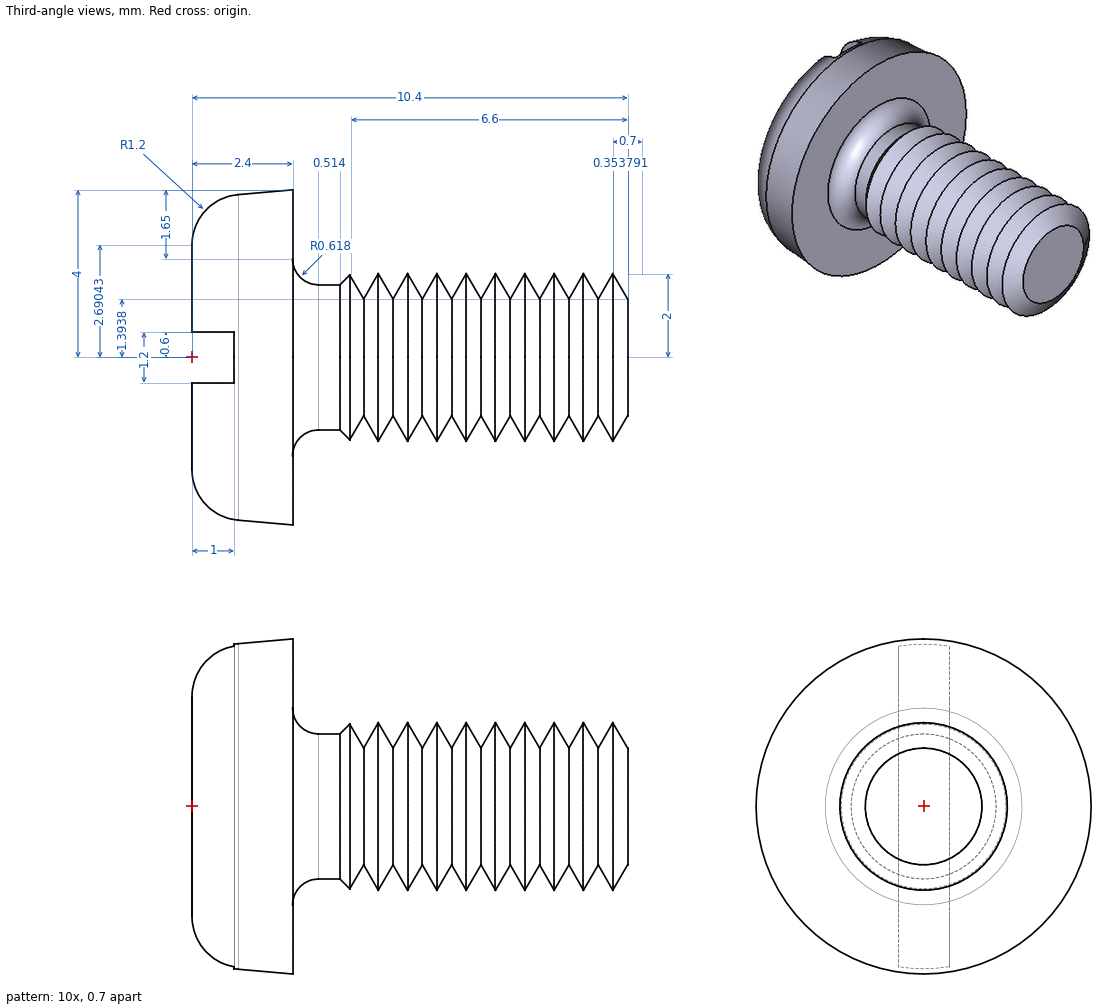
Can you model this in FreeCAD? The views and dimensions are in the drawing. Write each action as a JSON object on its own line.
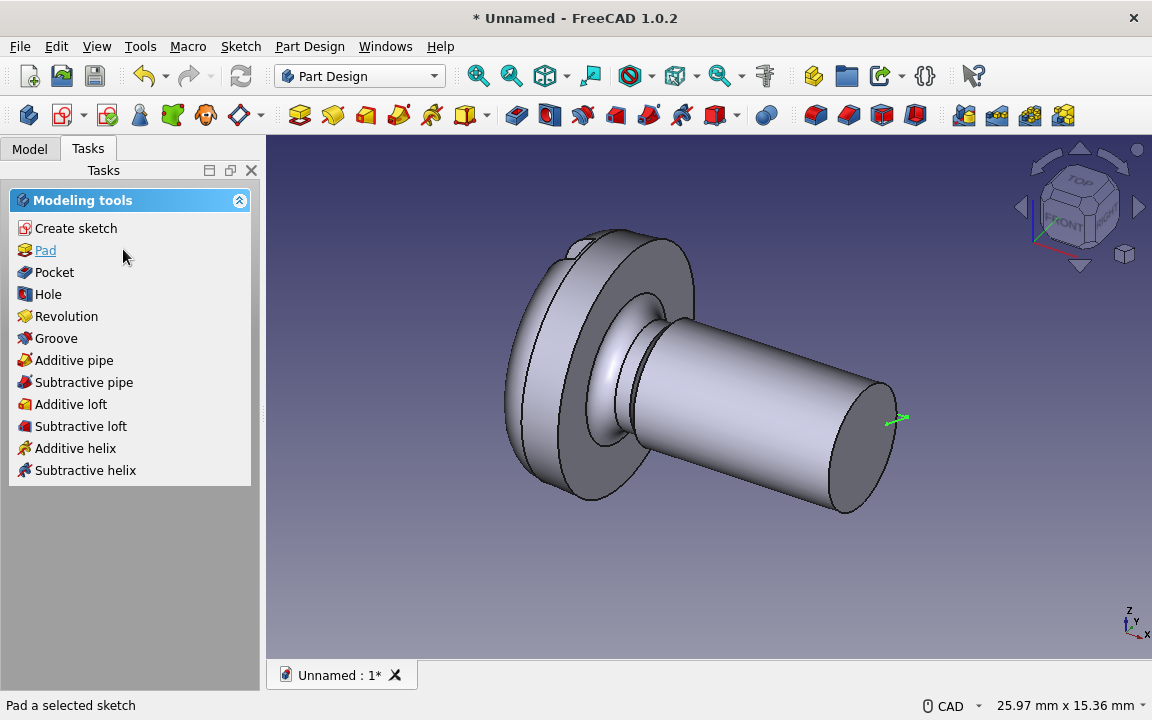
{"action": "left_click", "coordinate": [583, 116]}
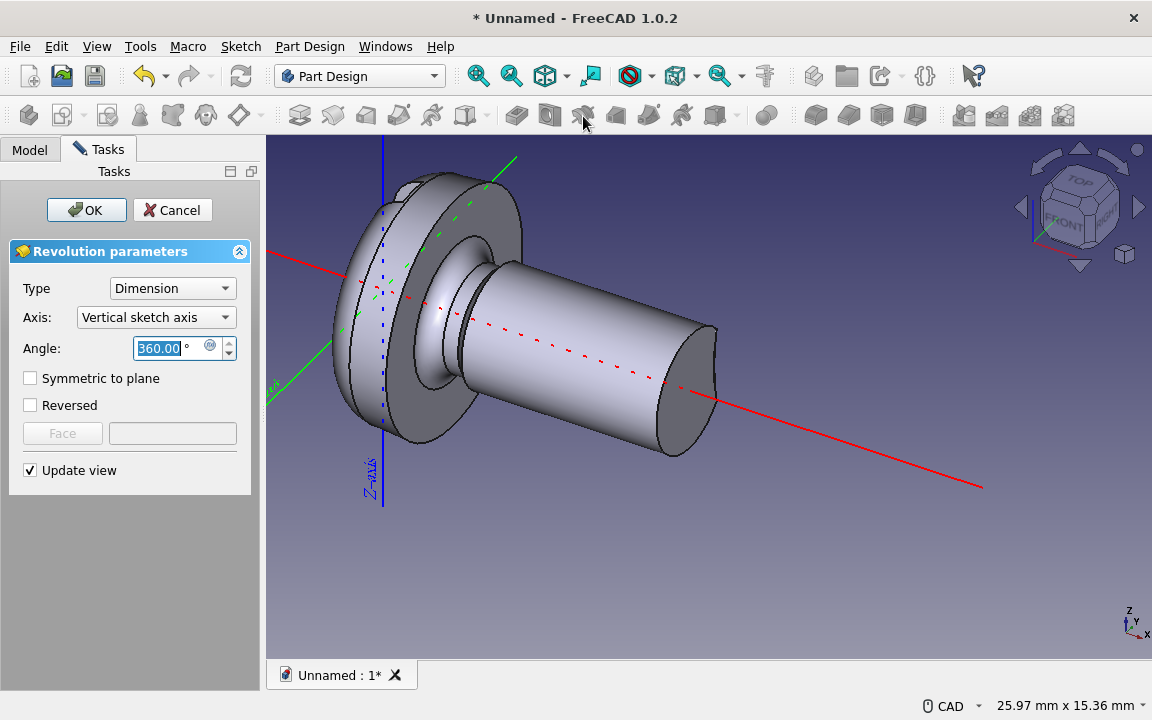
{"action": "left_click", "coordinate": [157, 318]}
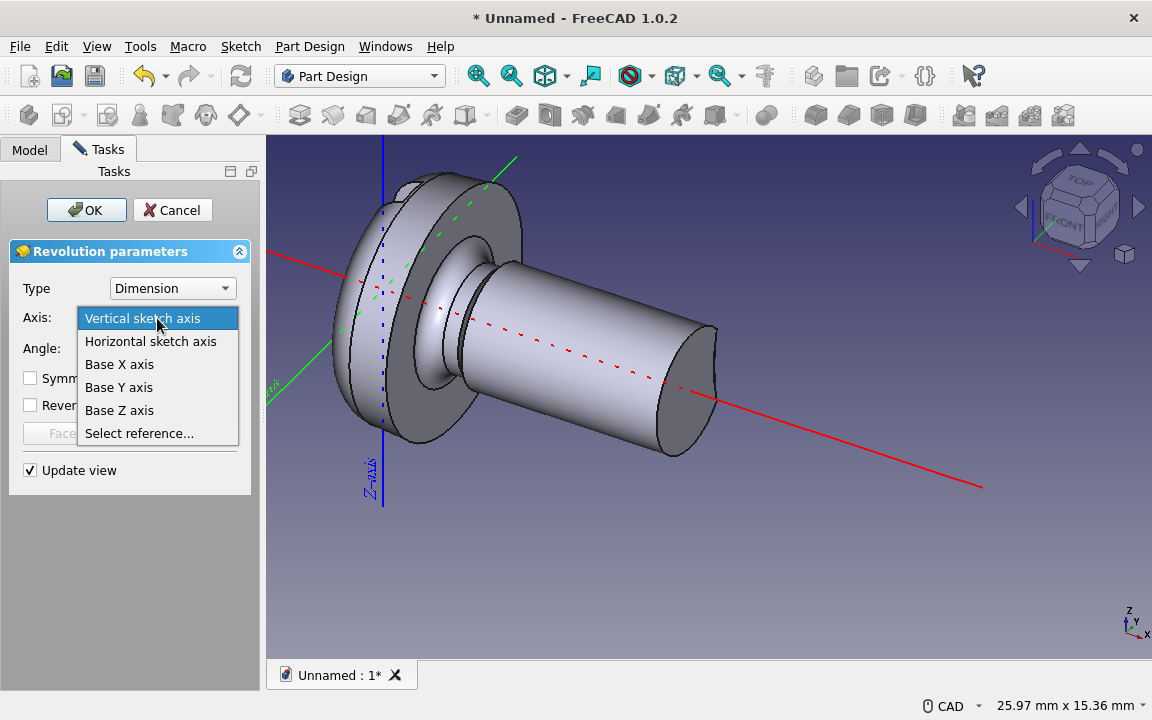
{"action": "left_click", "coordinate": [156, 342]}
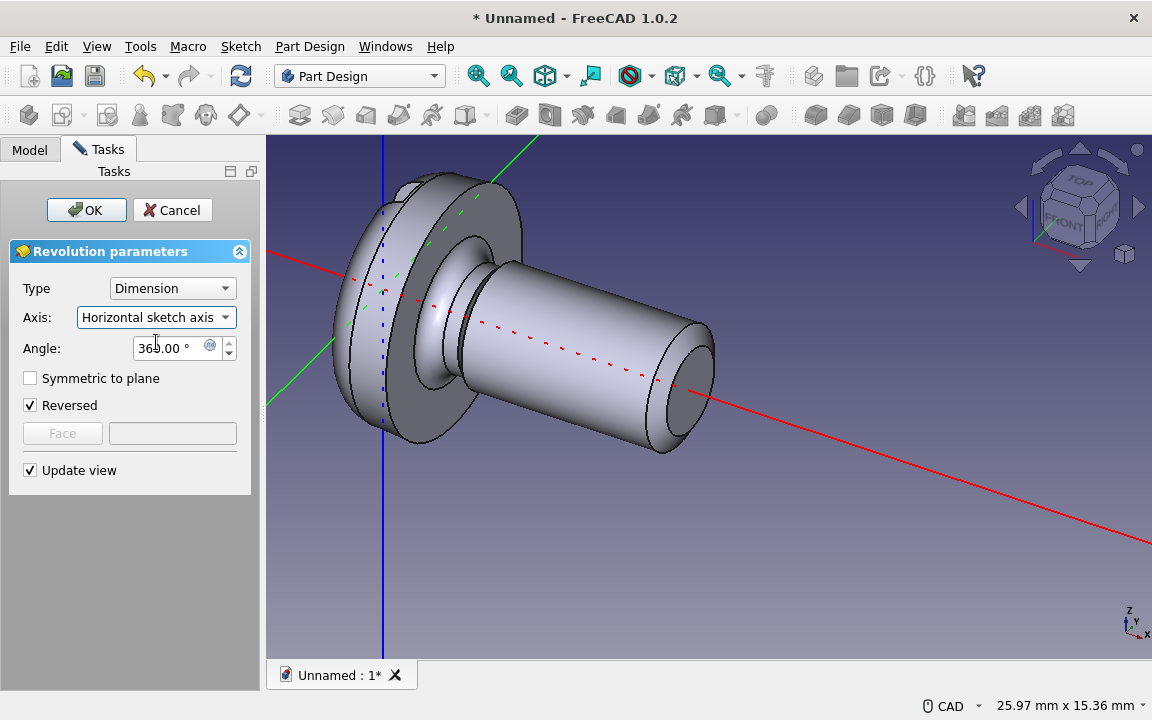
{"action": "left_click", "coordinate": [87, 210]}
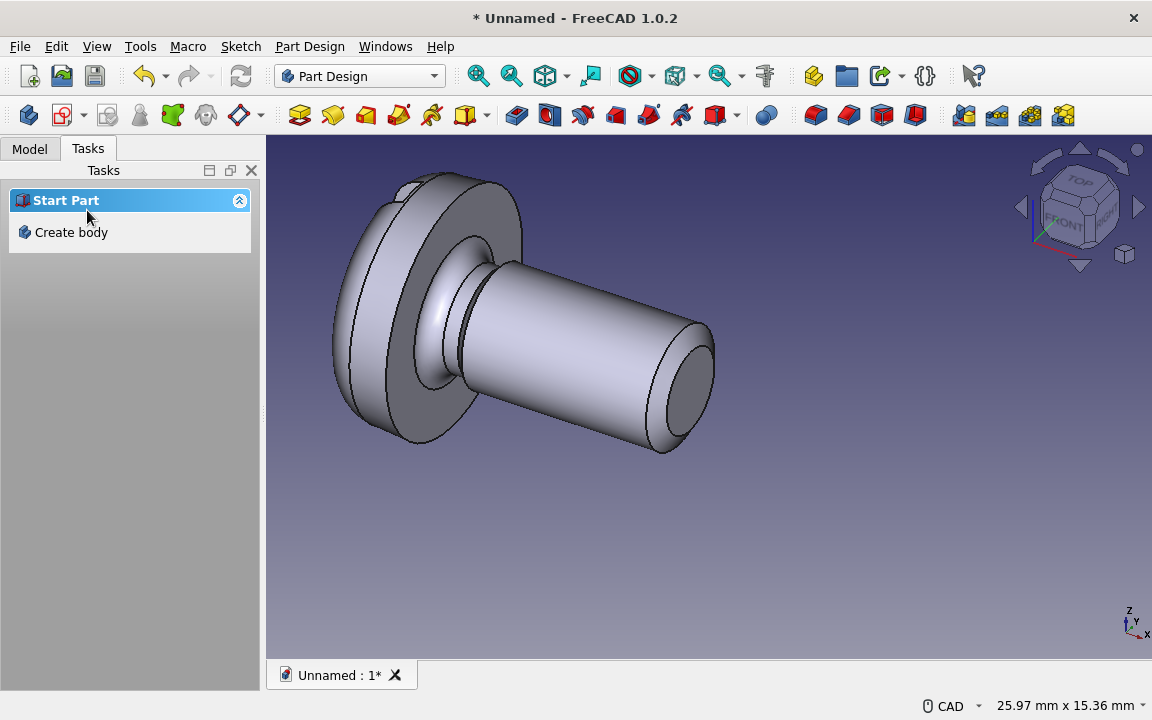
{"action": "left_click", "coordinate": [479, 76]}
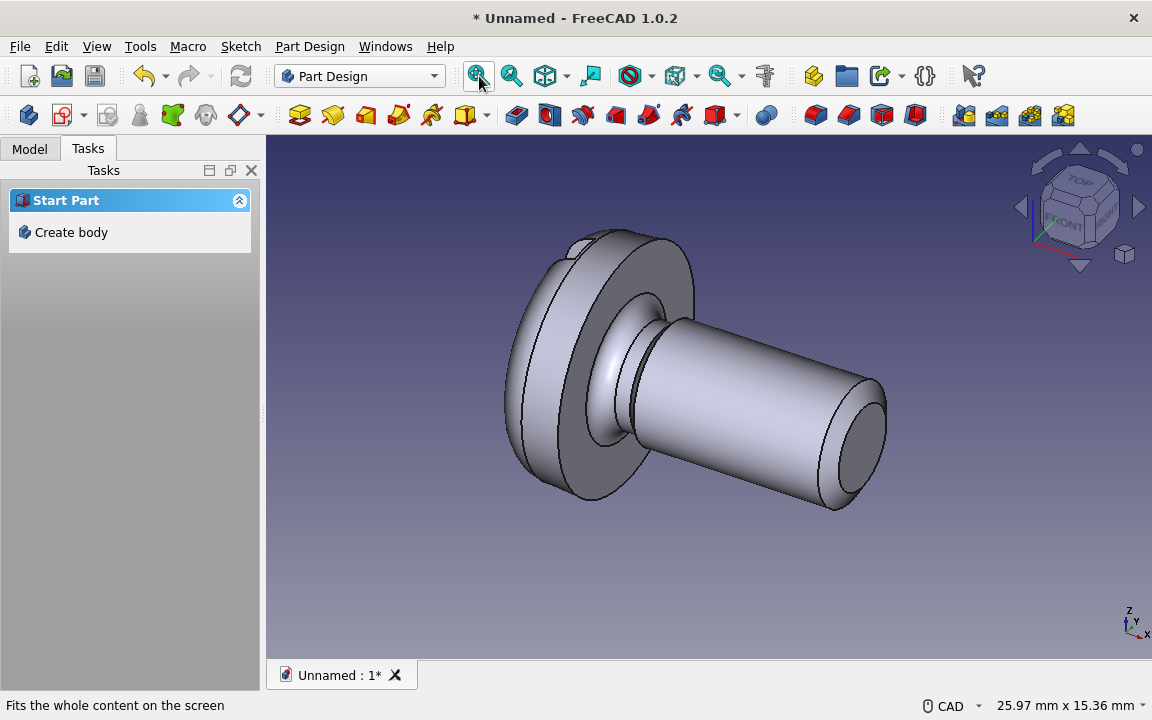
{"action": "left_click", "coordinate": [30, 148]}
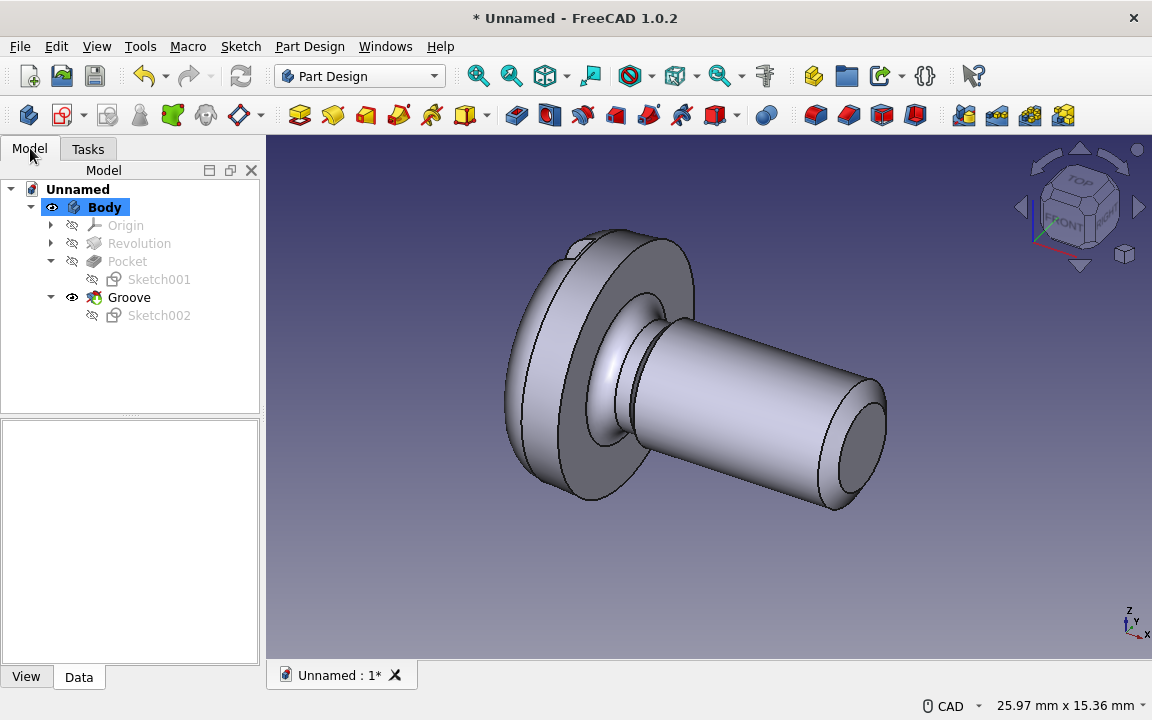
{"action": "left_click", "coordinate": [117, 297]}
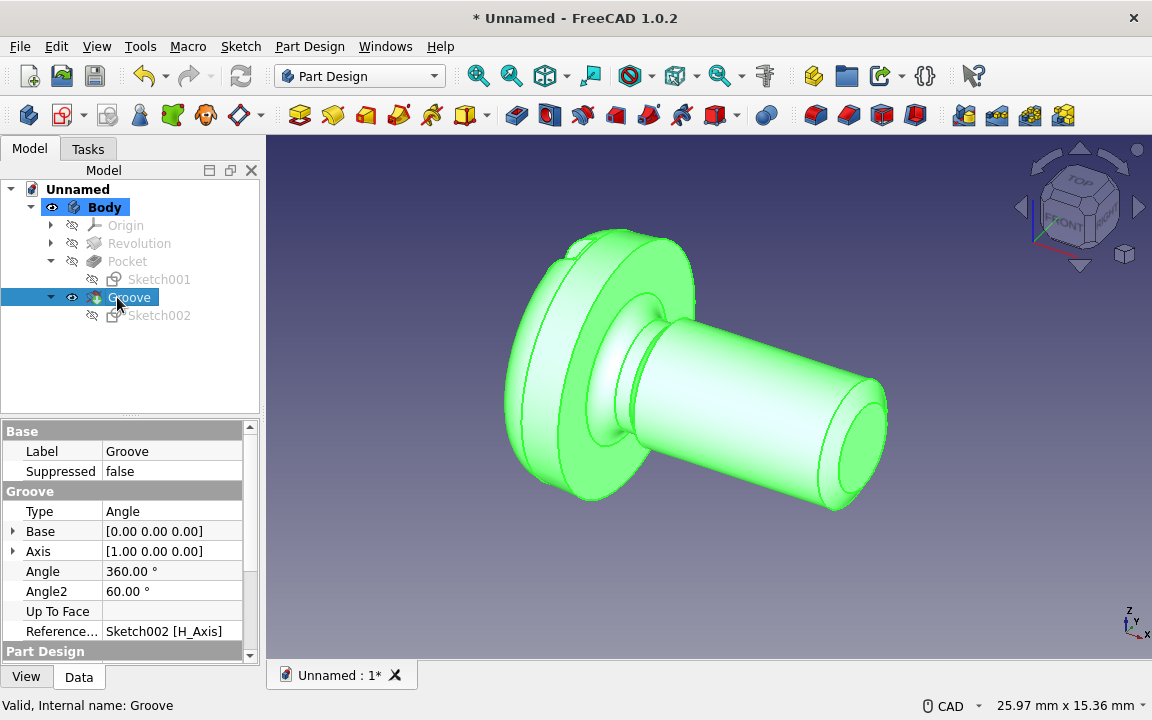
{"action": "left_click", "coordinate": [997, 116]}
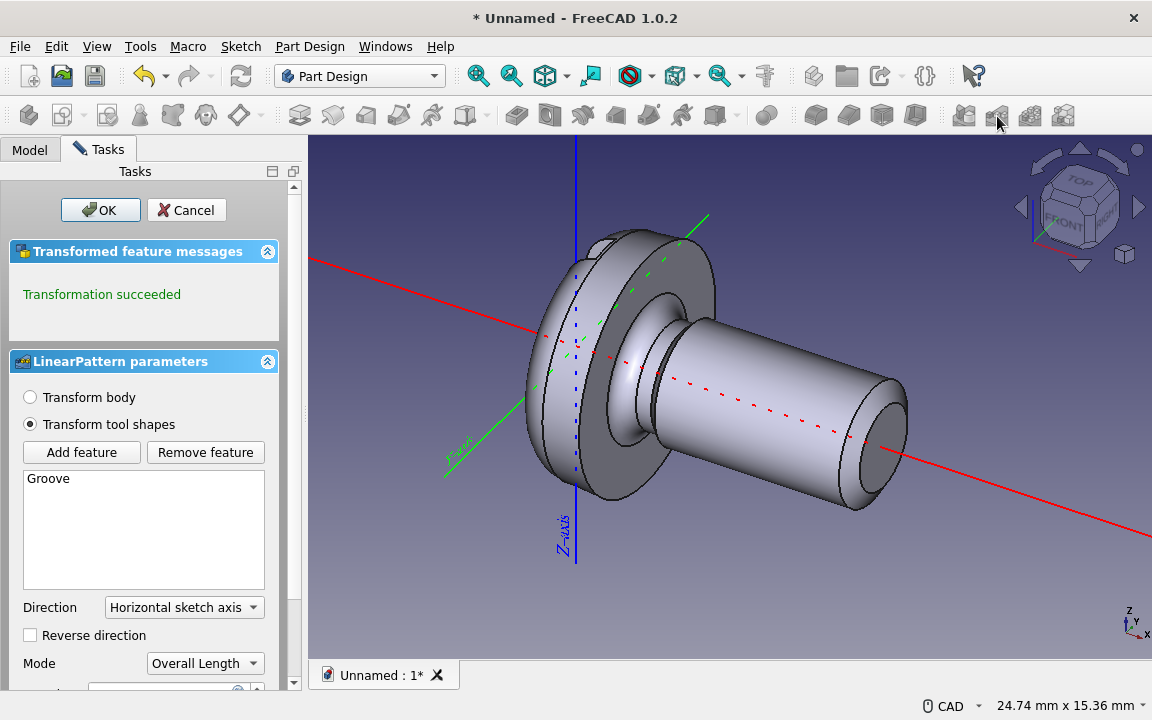
{"action": "left_click", "coordinate": [185, 608]}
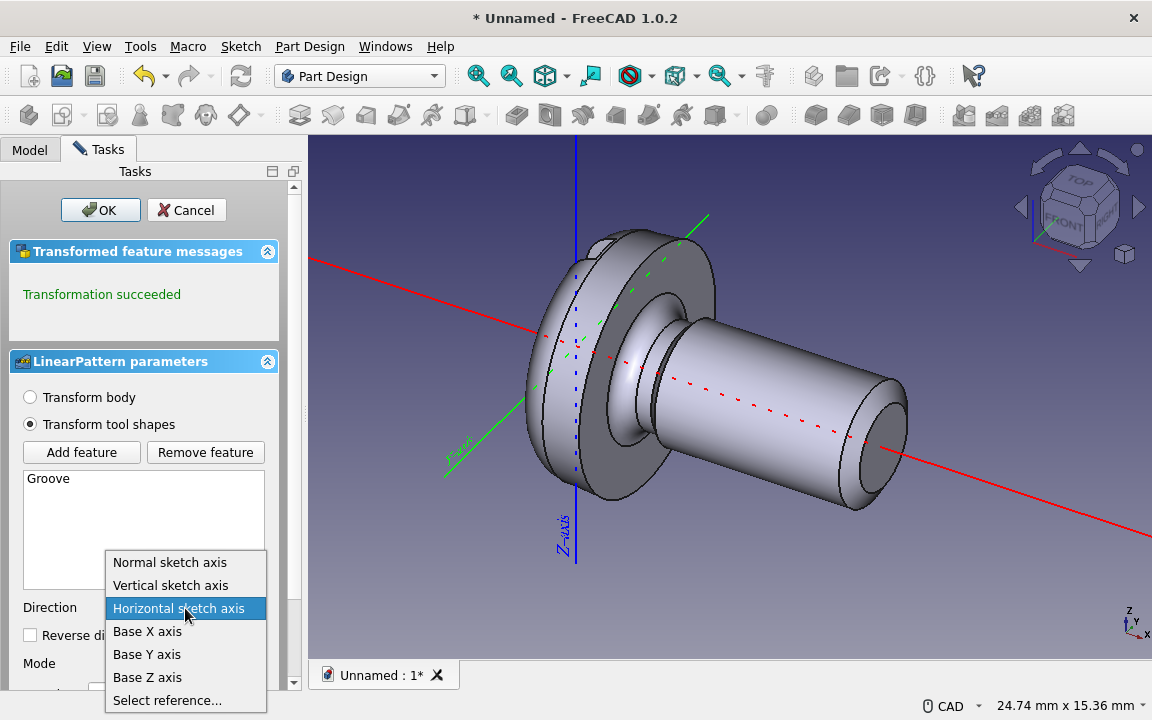
{"action": "left_click", "coordinate": [184, 632]}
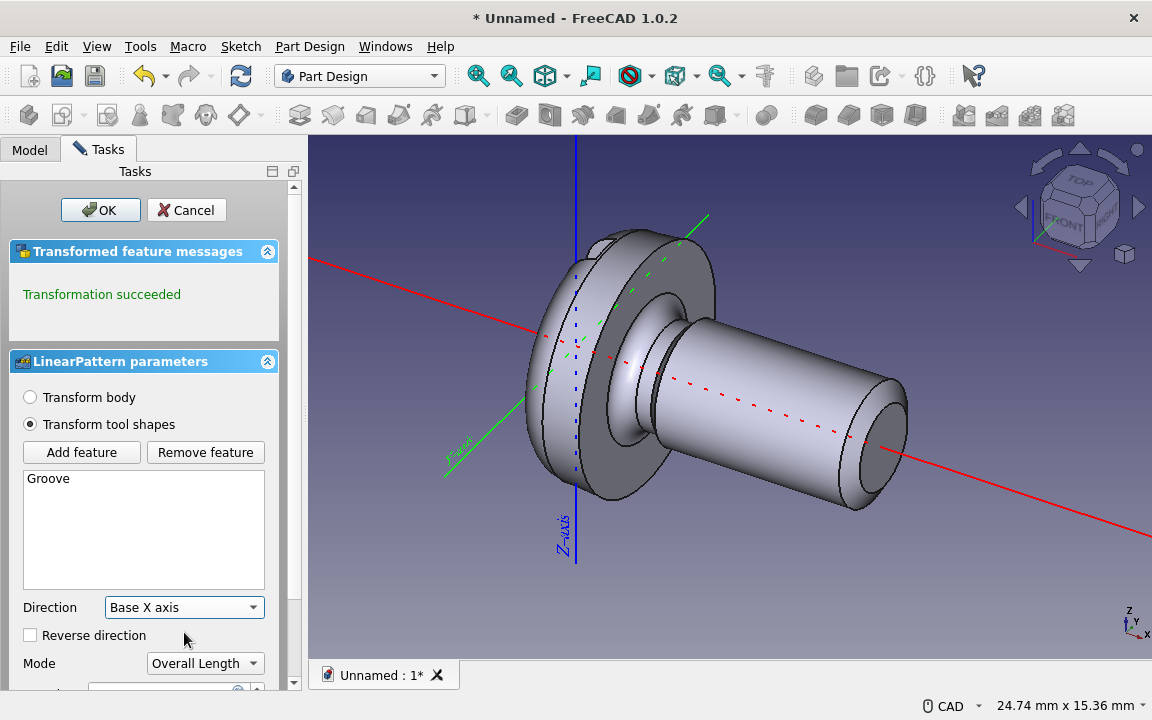
{"action": "left_click", "coordinate": [206, 664]}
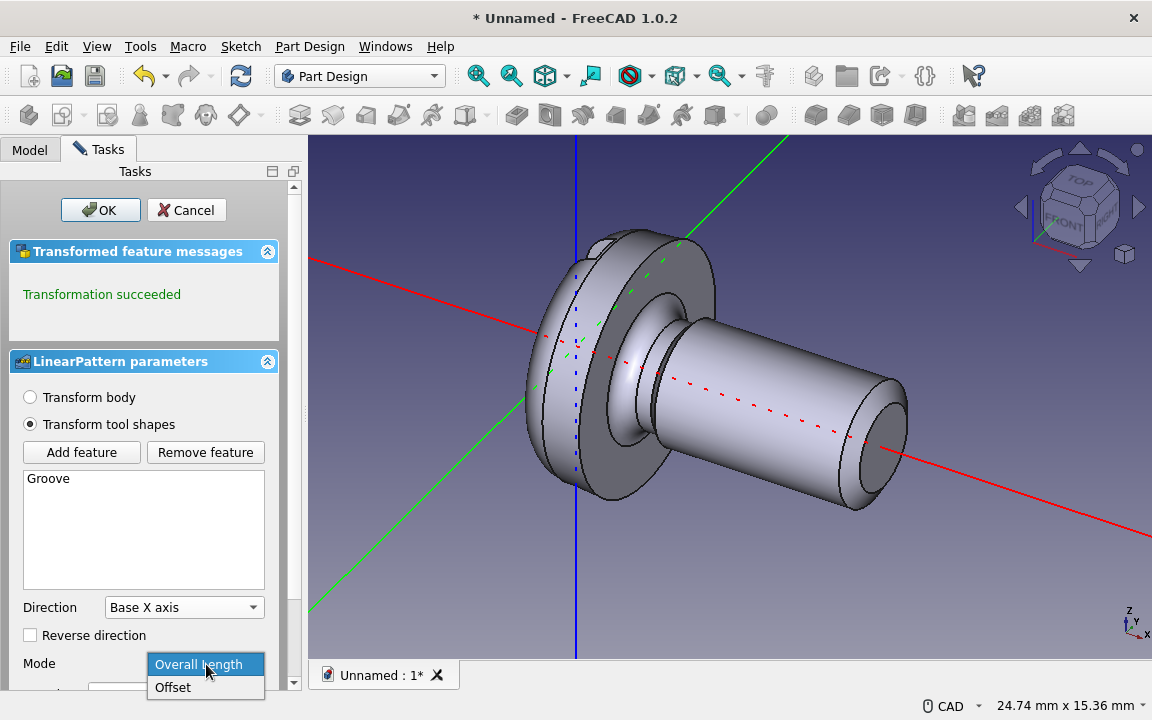
{"action": "left_click", "coordinate": [204, 688]}